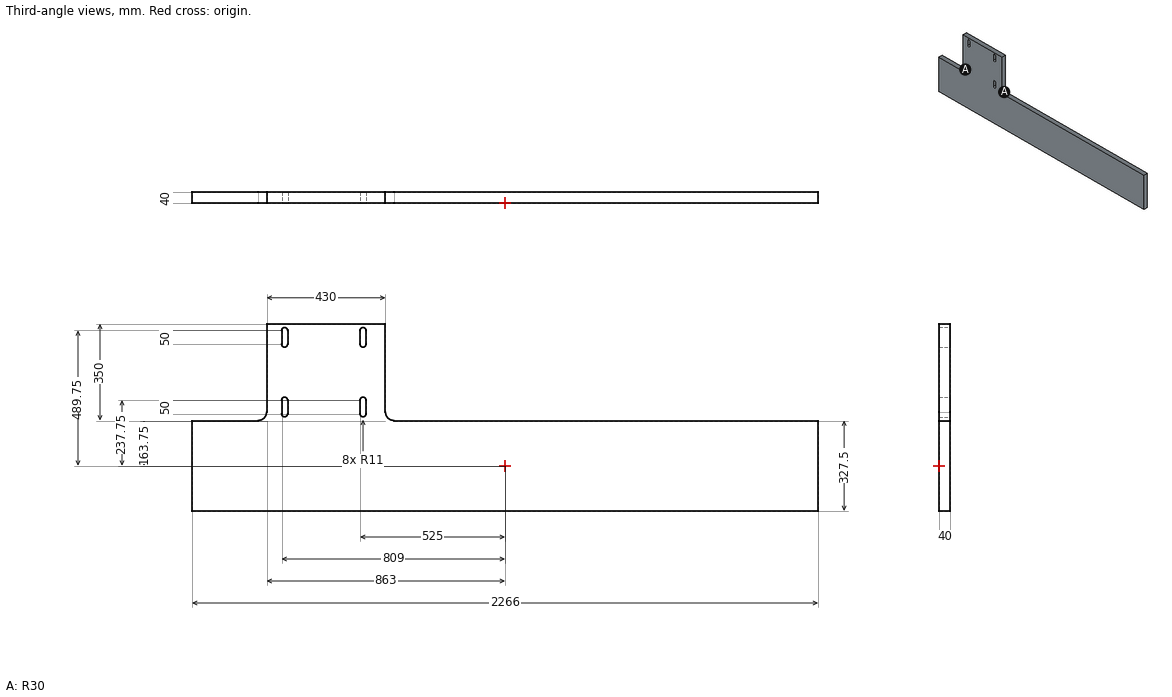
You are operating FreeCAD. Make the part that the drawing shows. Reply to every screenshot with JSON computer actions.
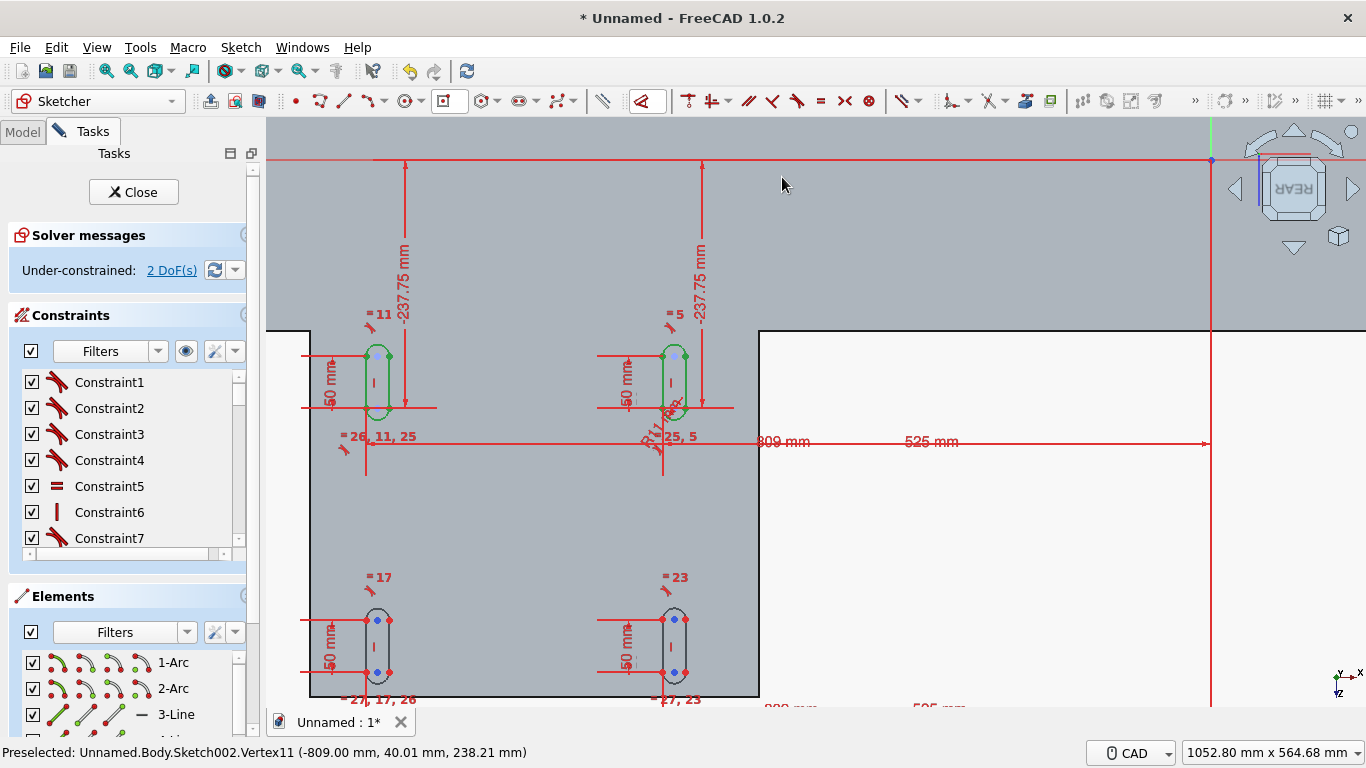
{"action": "left_click", "coordinate": [366, 672]}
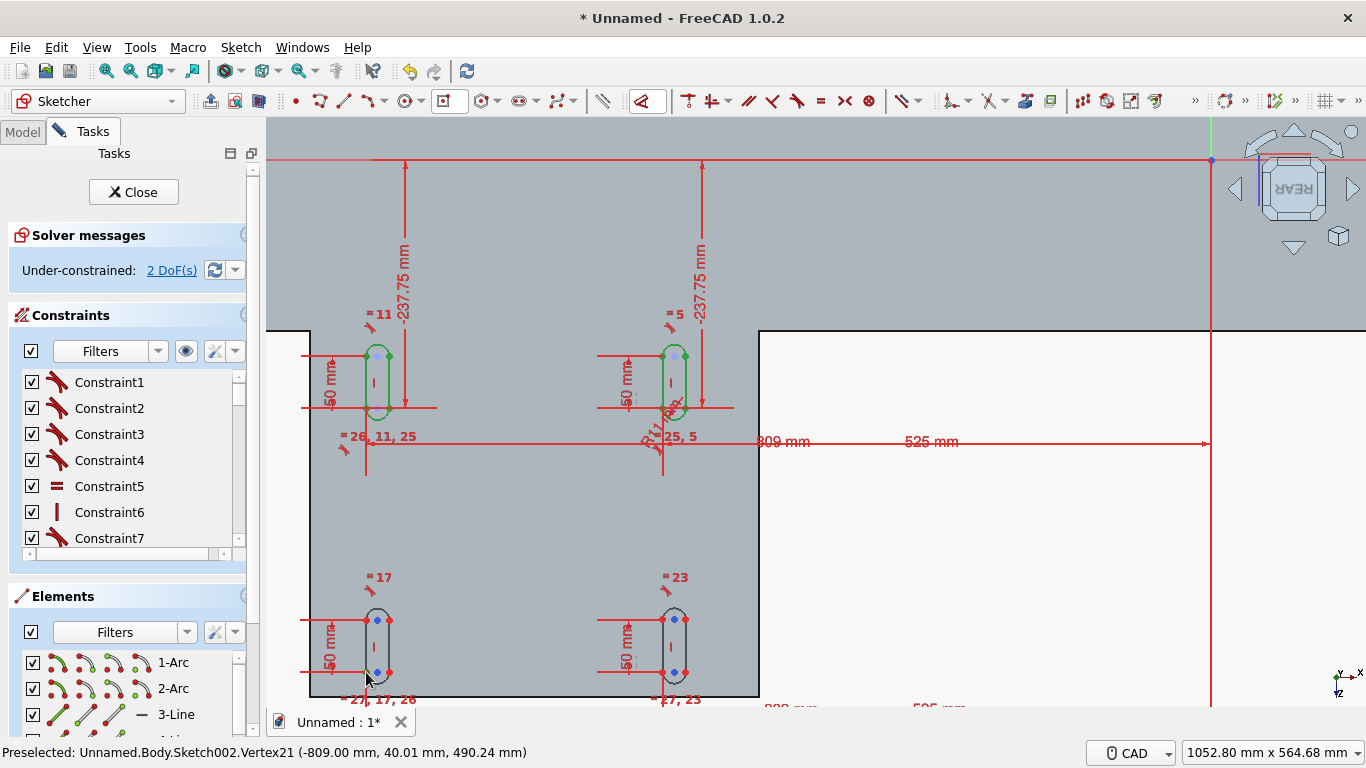
{"action": "key", "text": "i"}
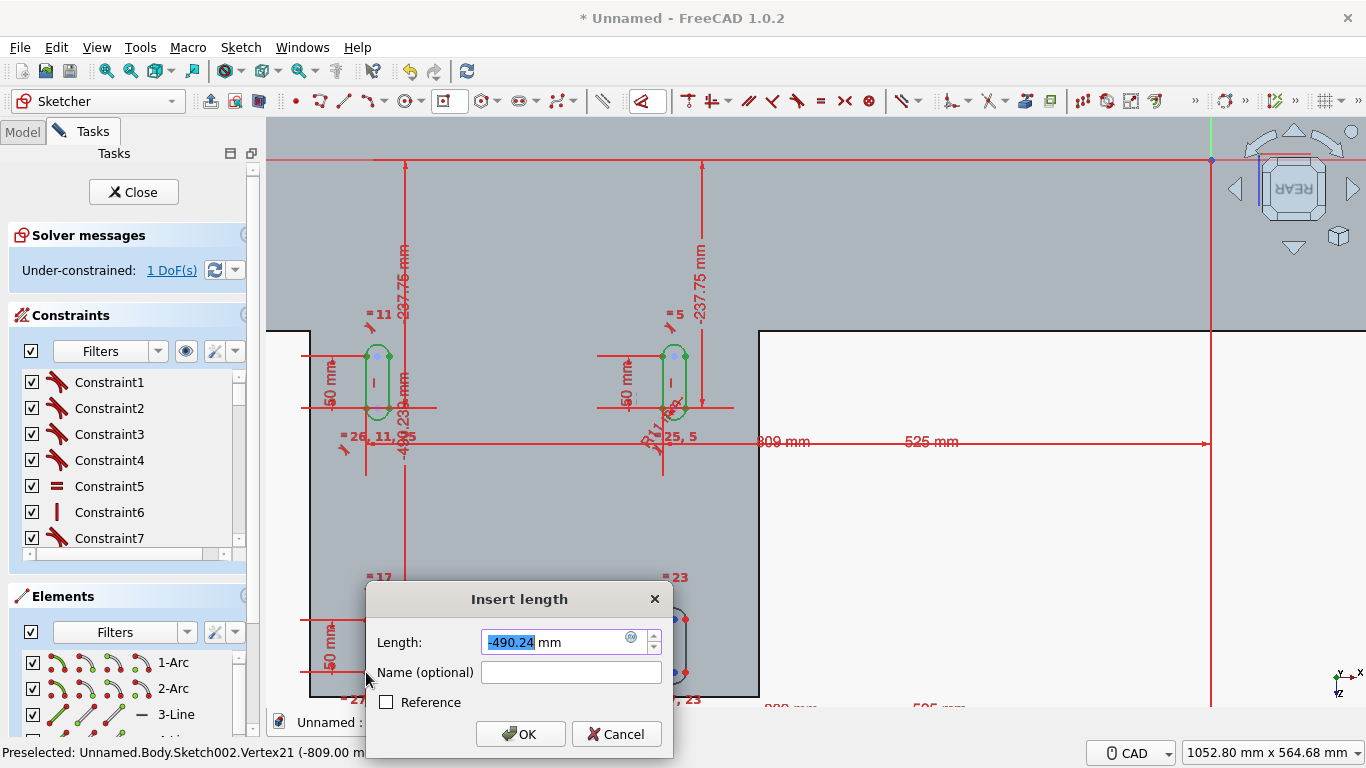
{"action": "type", "text": "-489.75"}
{"action": "key", "text": "Return"}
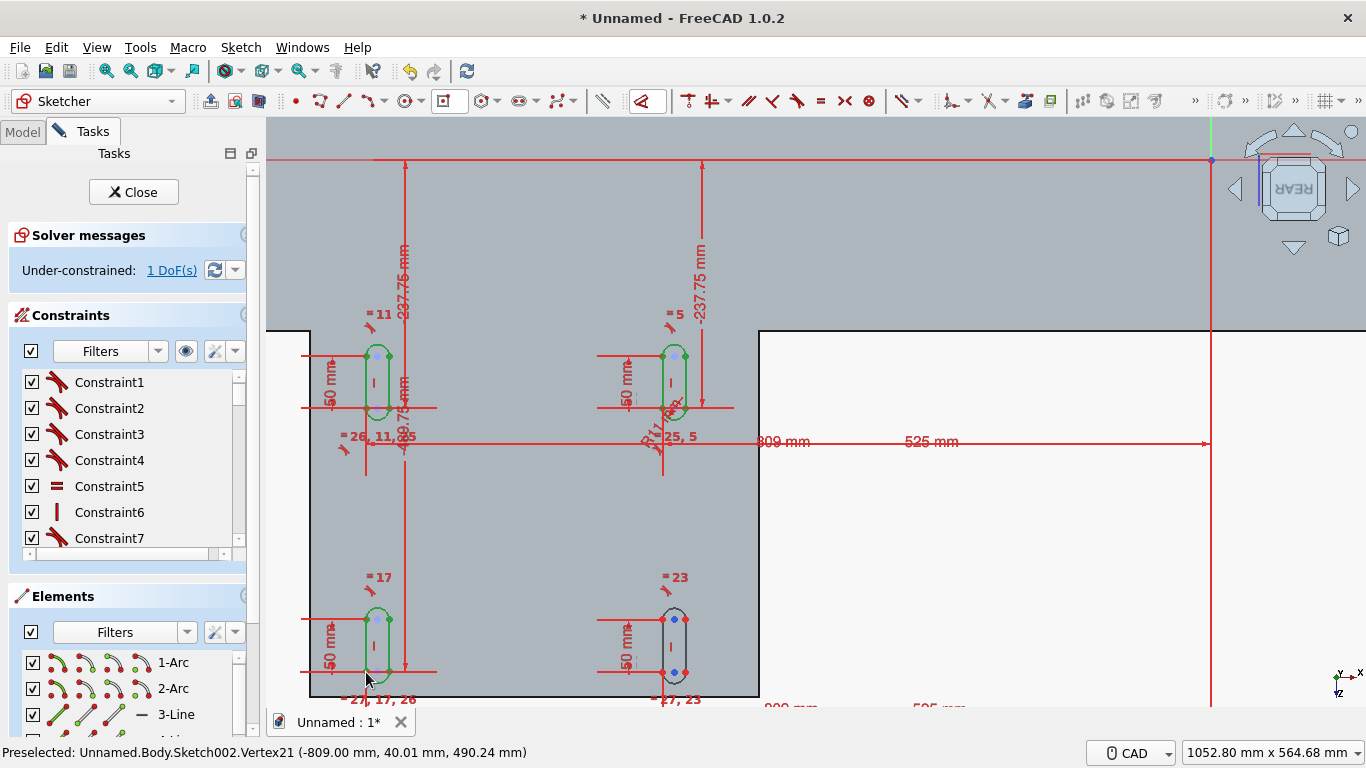
{"action": "left_click", "coordinate": [663, 672]}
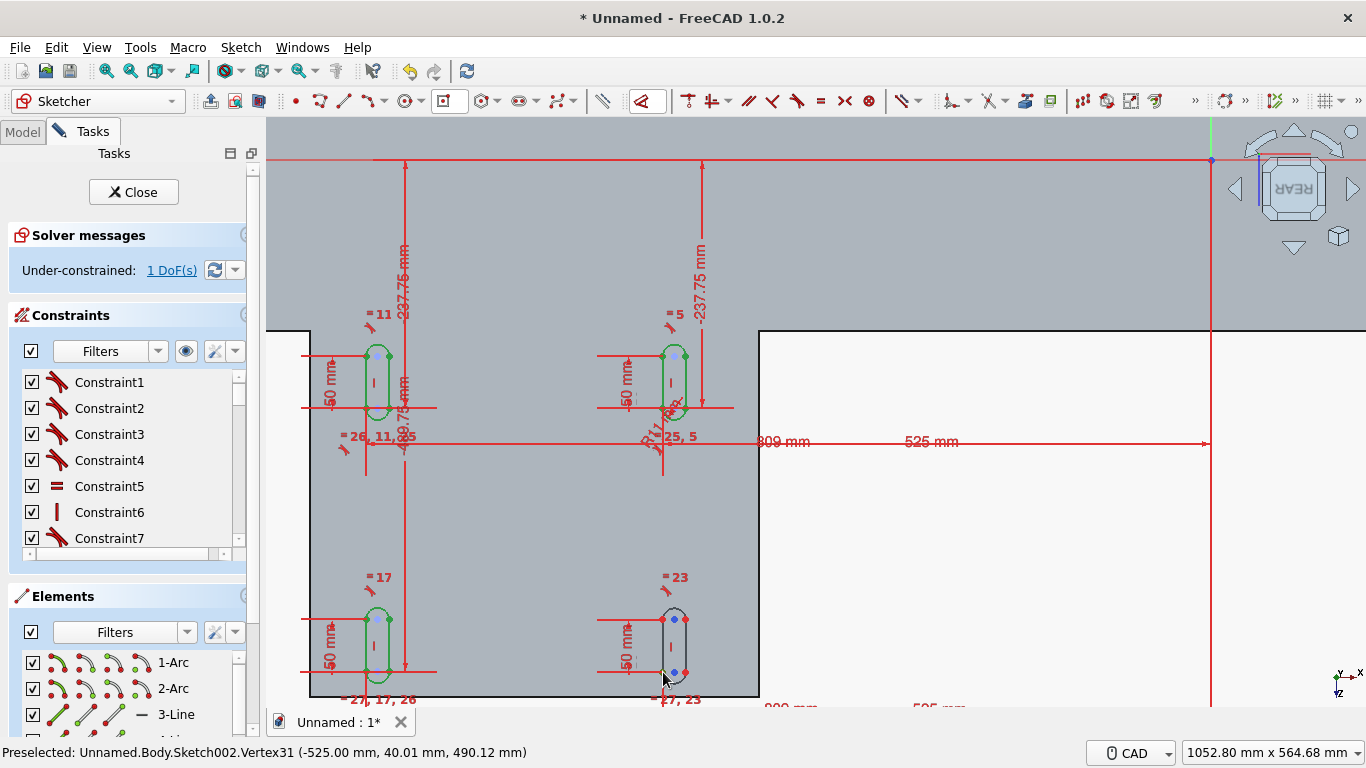
{"action": "left_click", "coordinate": [660, 102]}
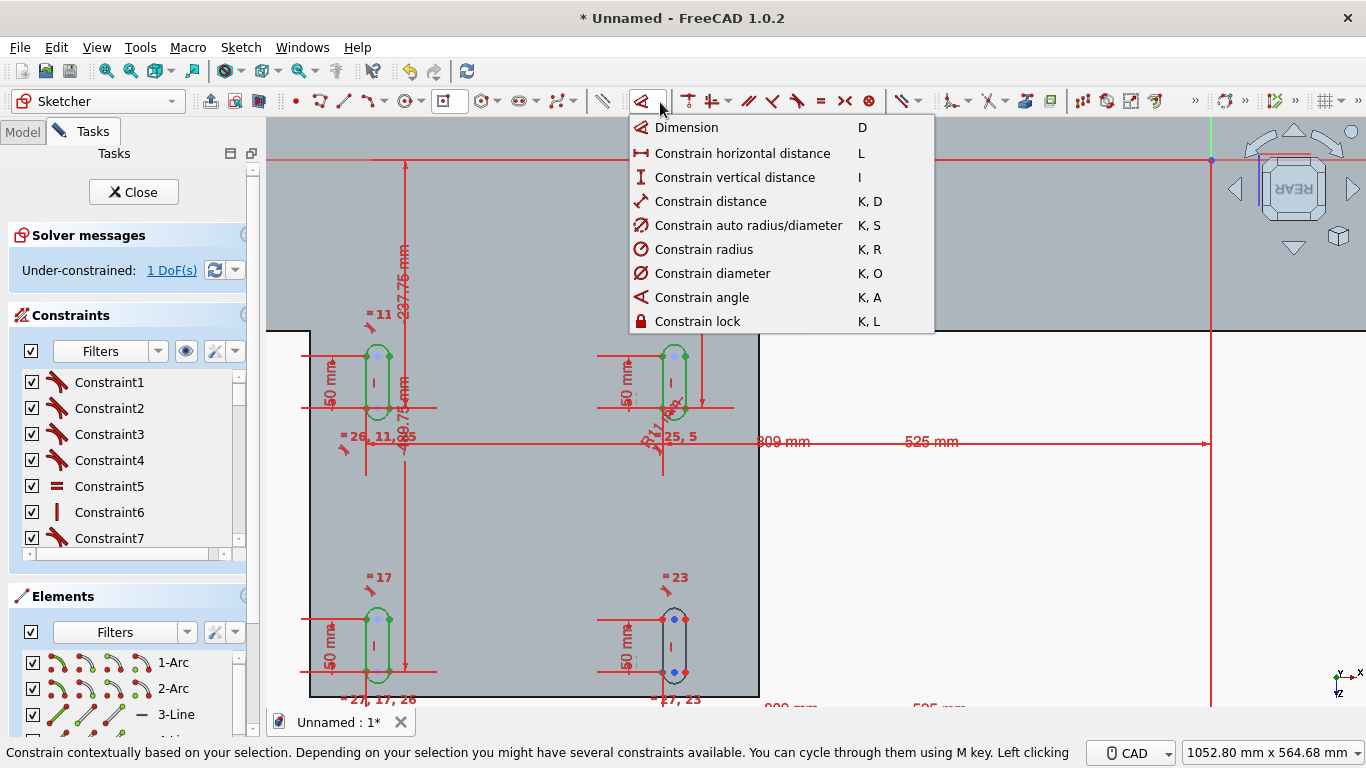
{"action": "left_click", "coordinate": [782, 177]}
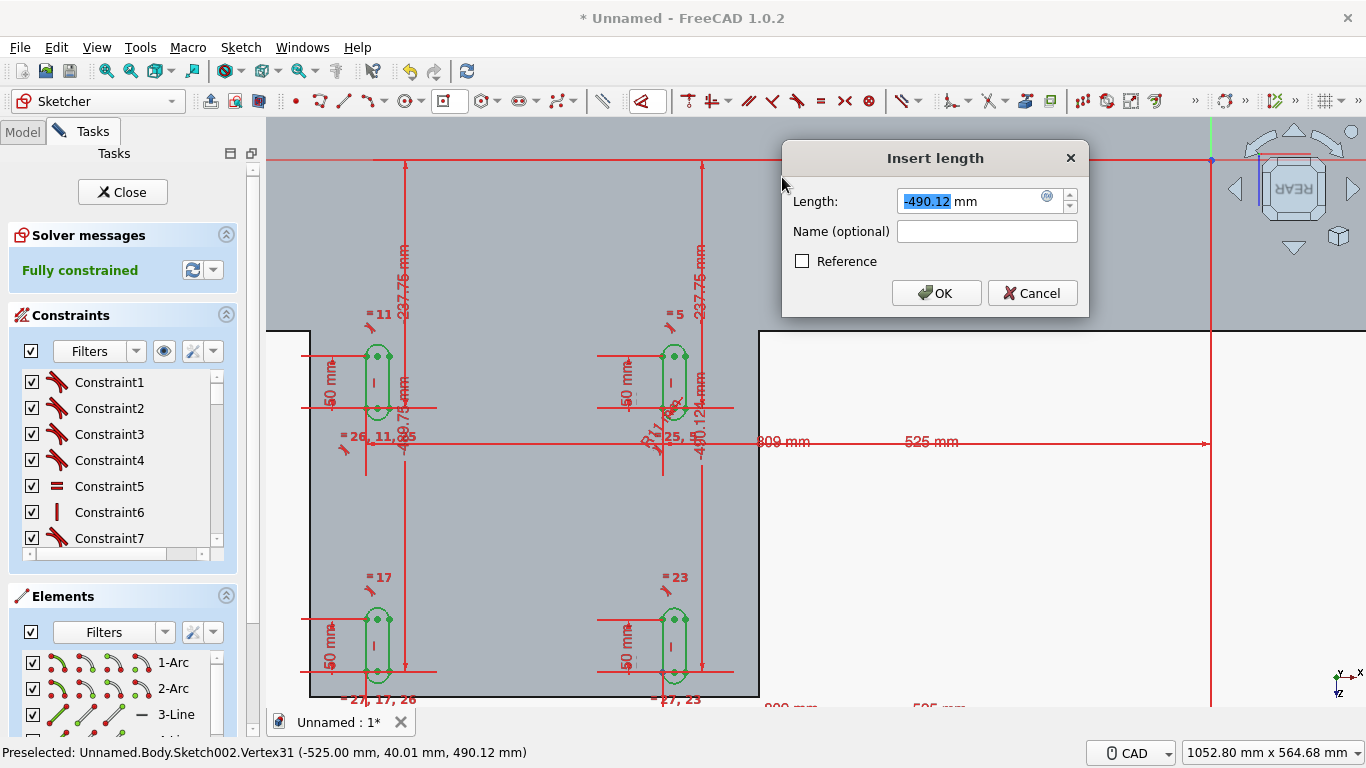
{"action": "type", "text": "-489.75"}
{"action": "key", "text": "Return"}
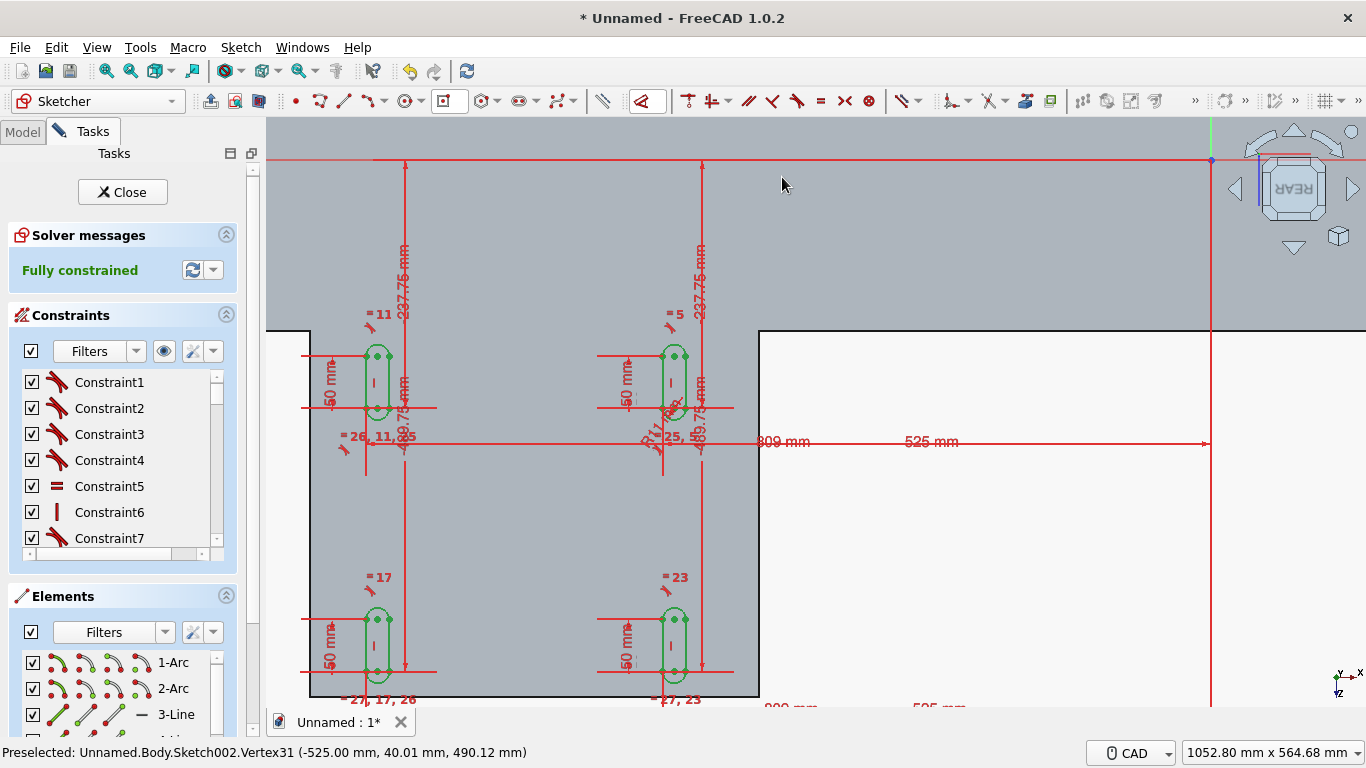
{"action": "left_click", "coordinate": [123, 192]}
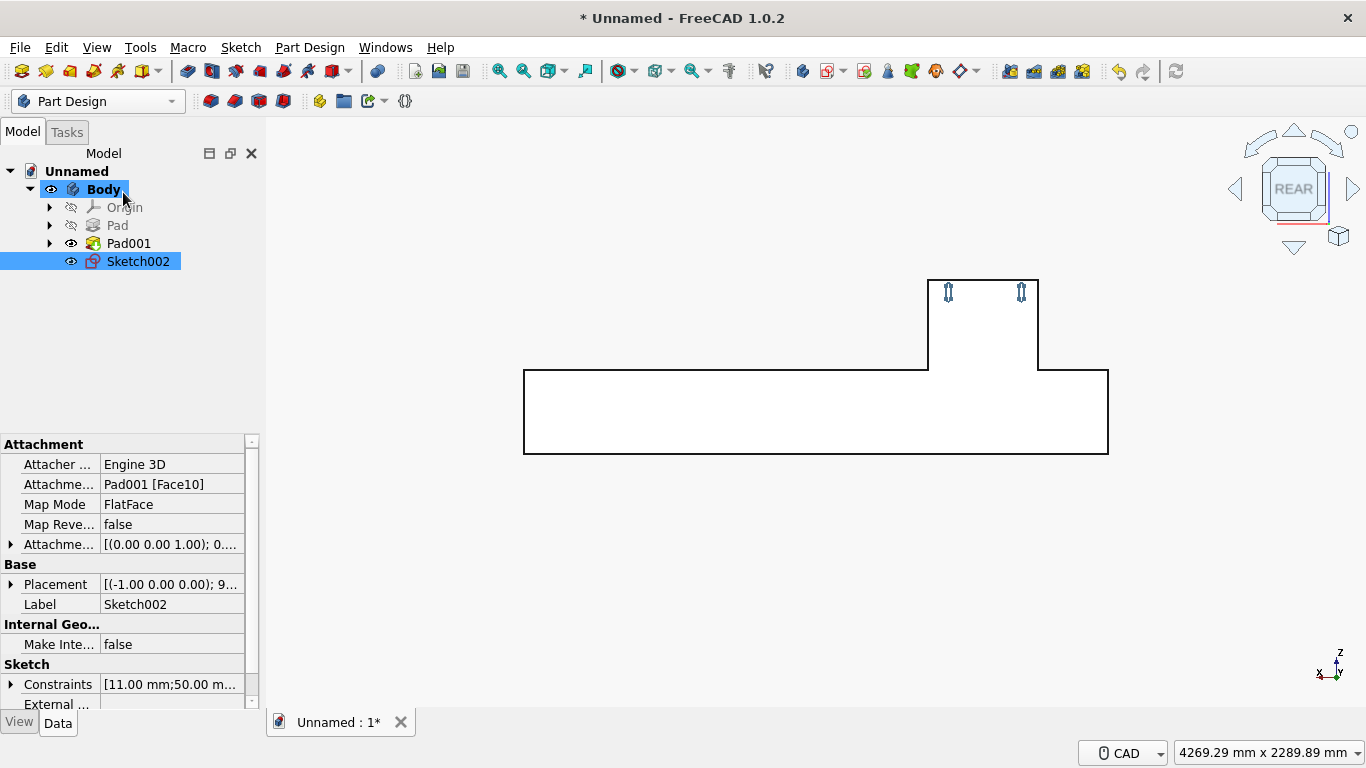
{"action": "left_click", "coordinate": [188, 72]}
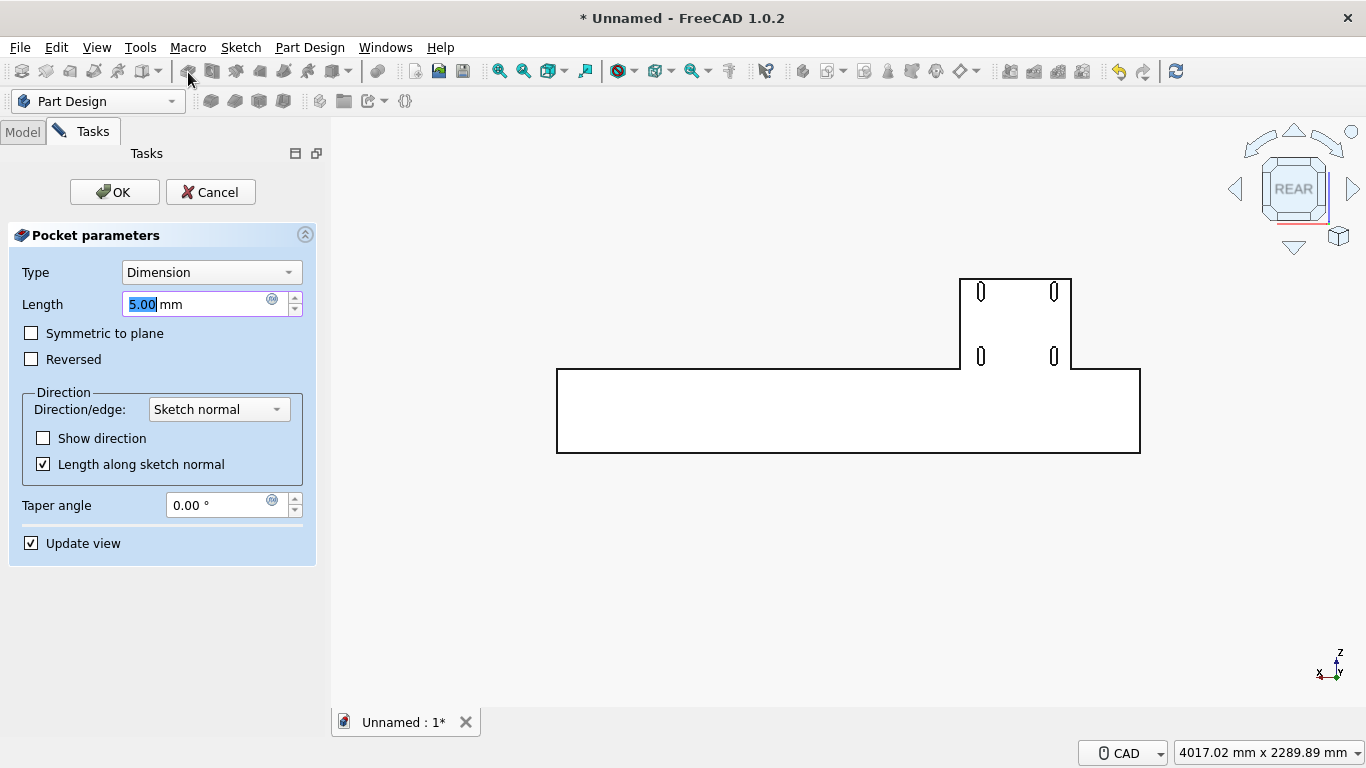
{"action": "left_click", "coordinate": [212, 272]}